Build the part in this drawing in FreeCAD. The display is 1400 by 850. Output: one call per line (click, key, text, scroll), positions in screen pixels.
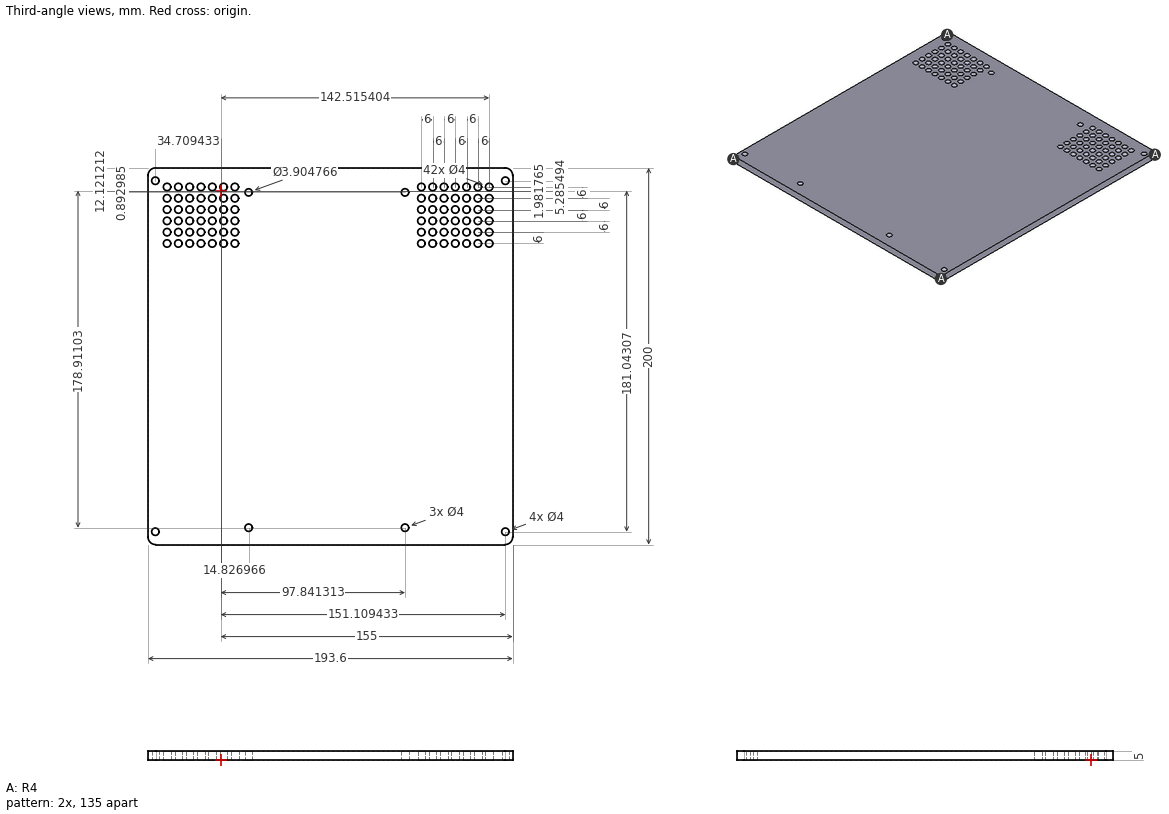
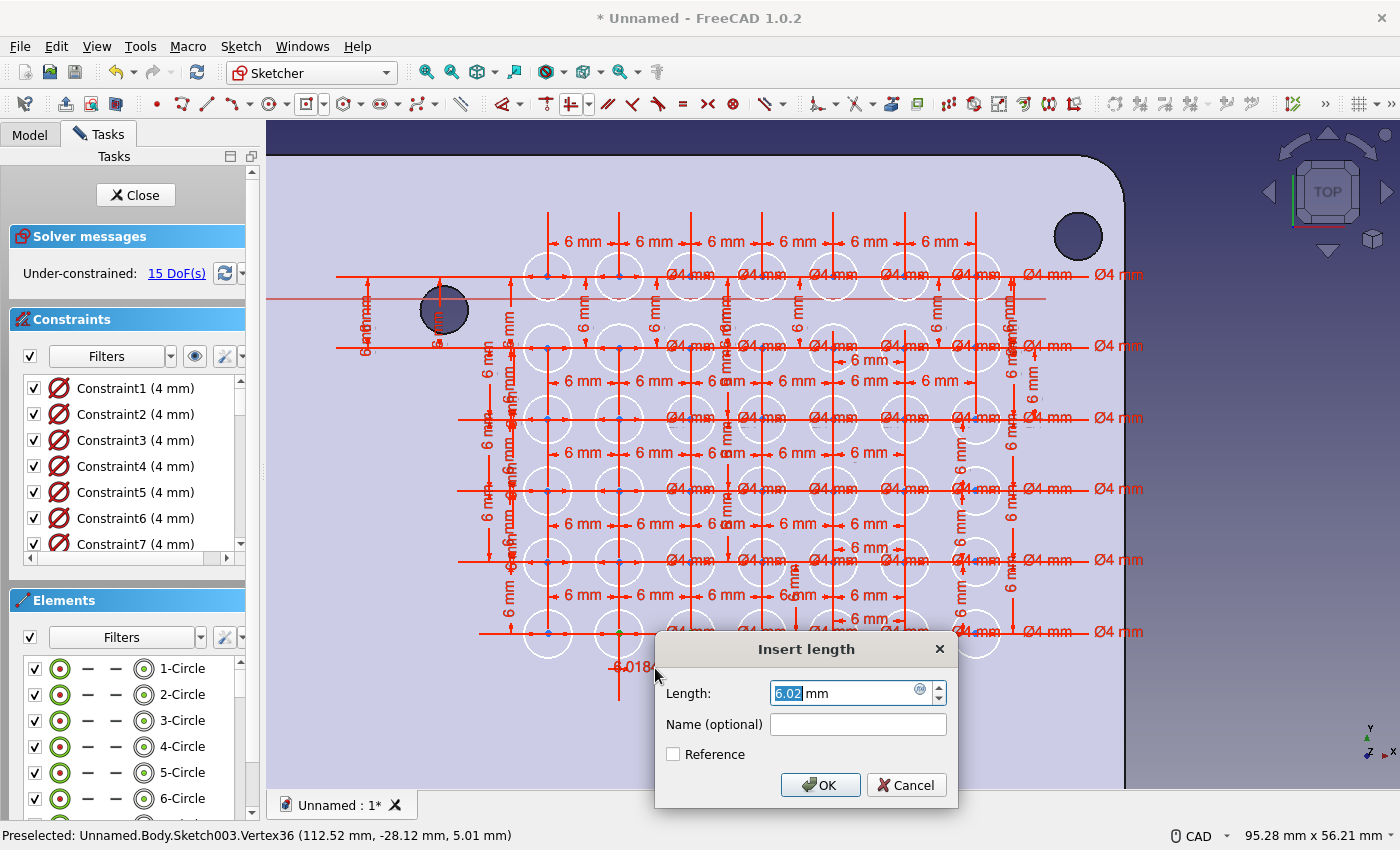
text(6)
key(Return)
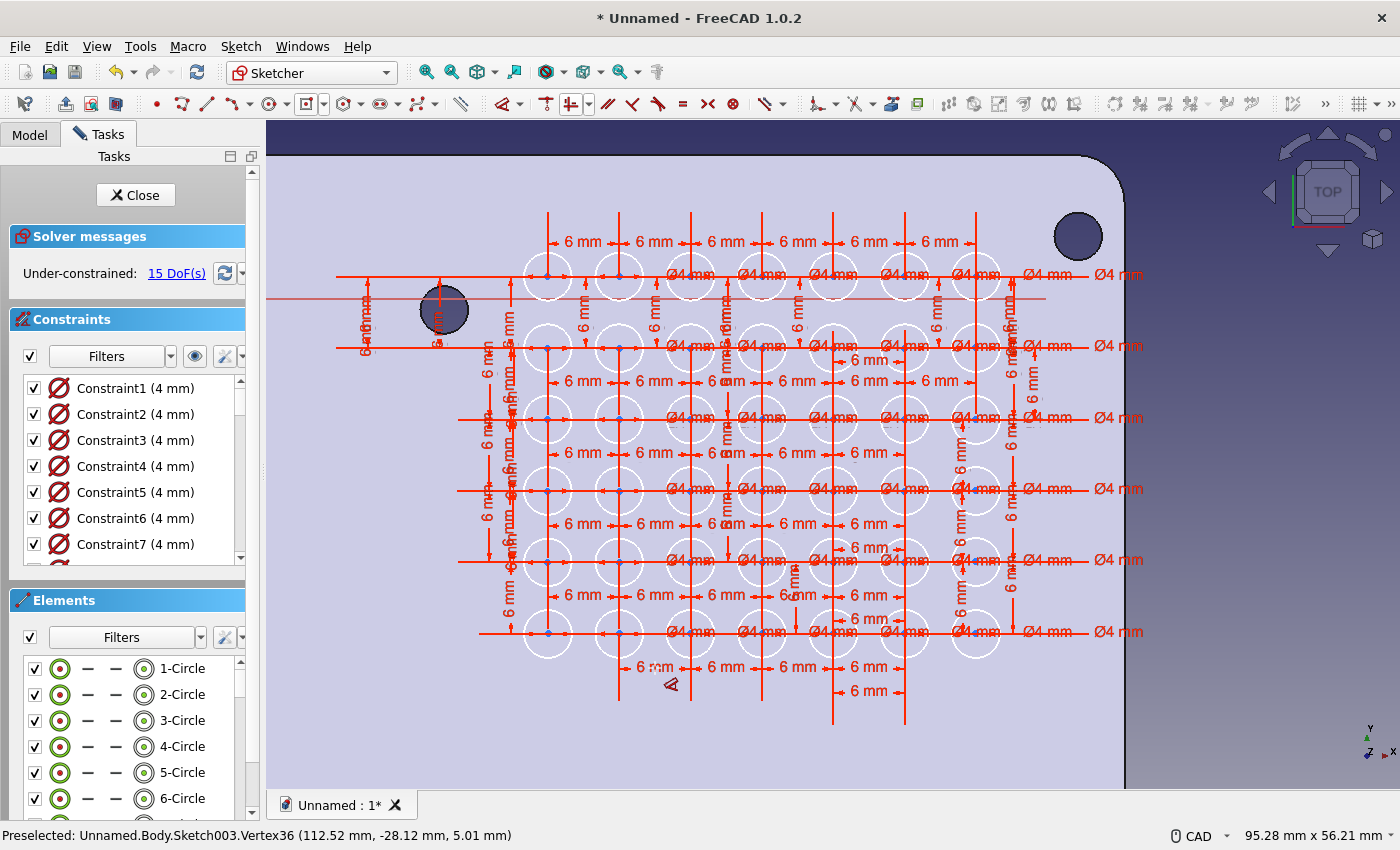
click(619, 562)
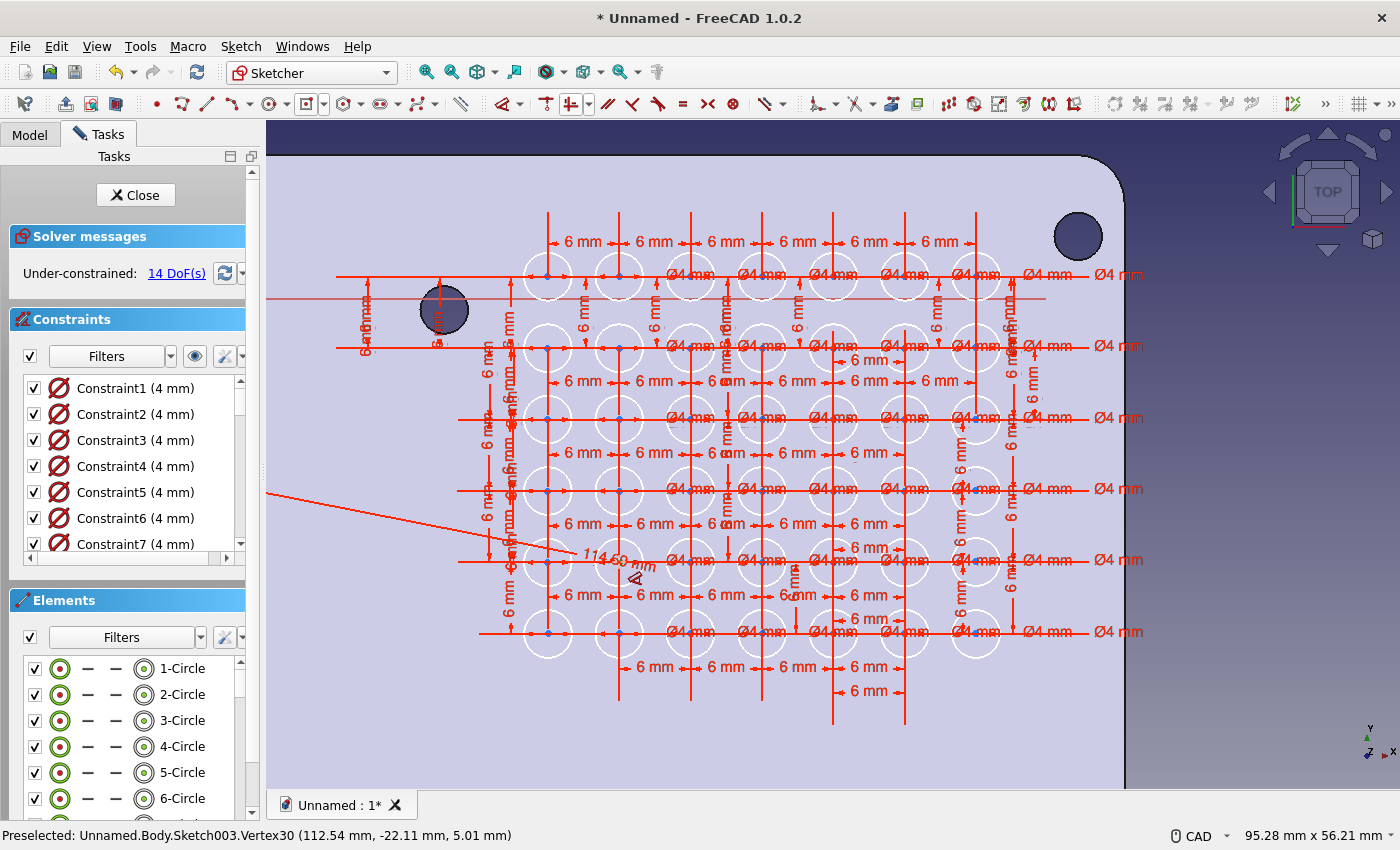
click(619, 634)
click(489, 573)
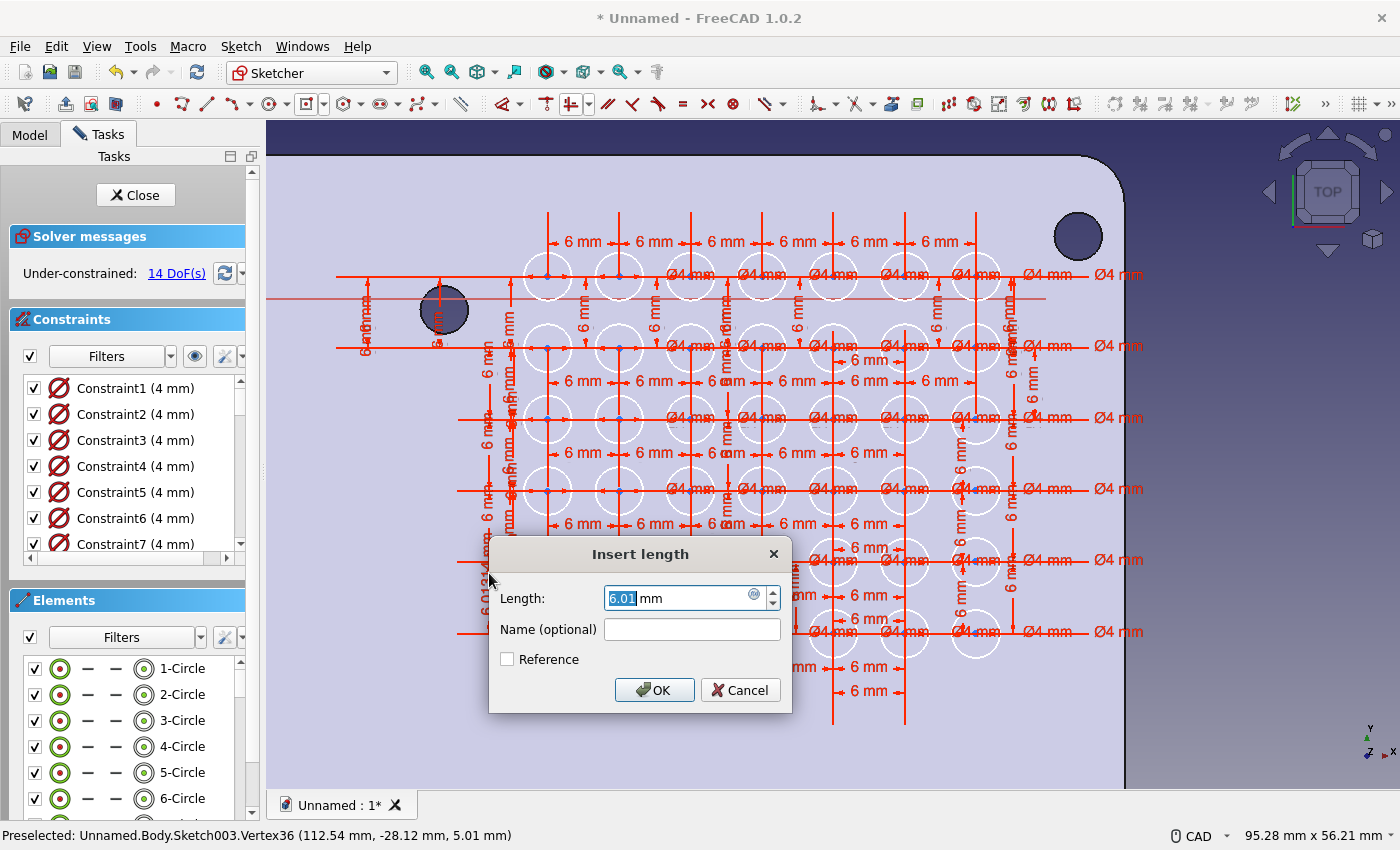
text(6)
key(Return)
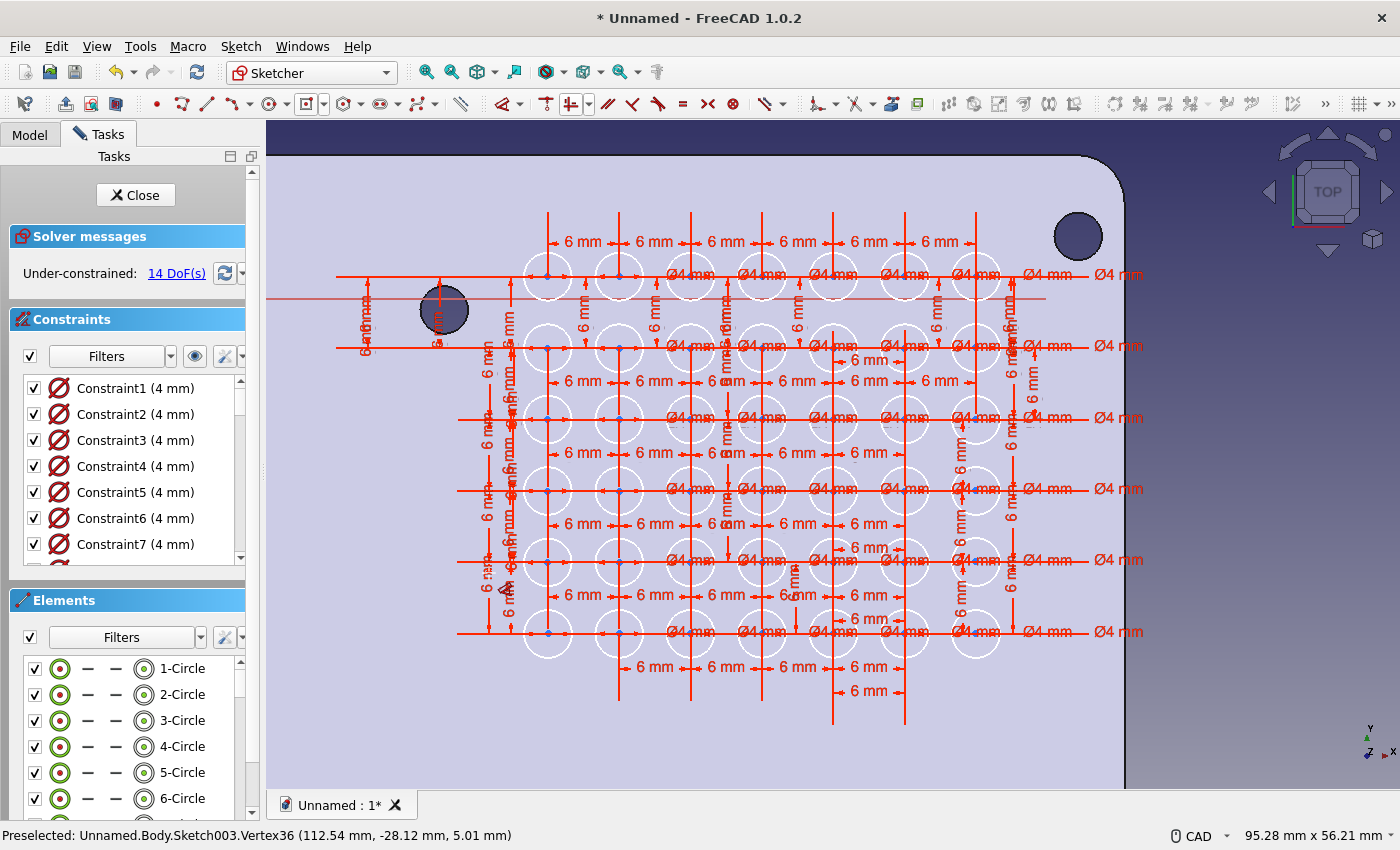
click(619, 634)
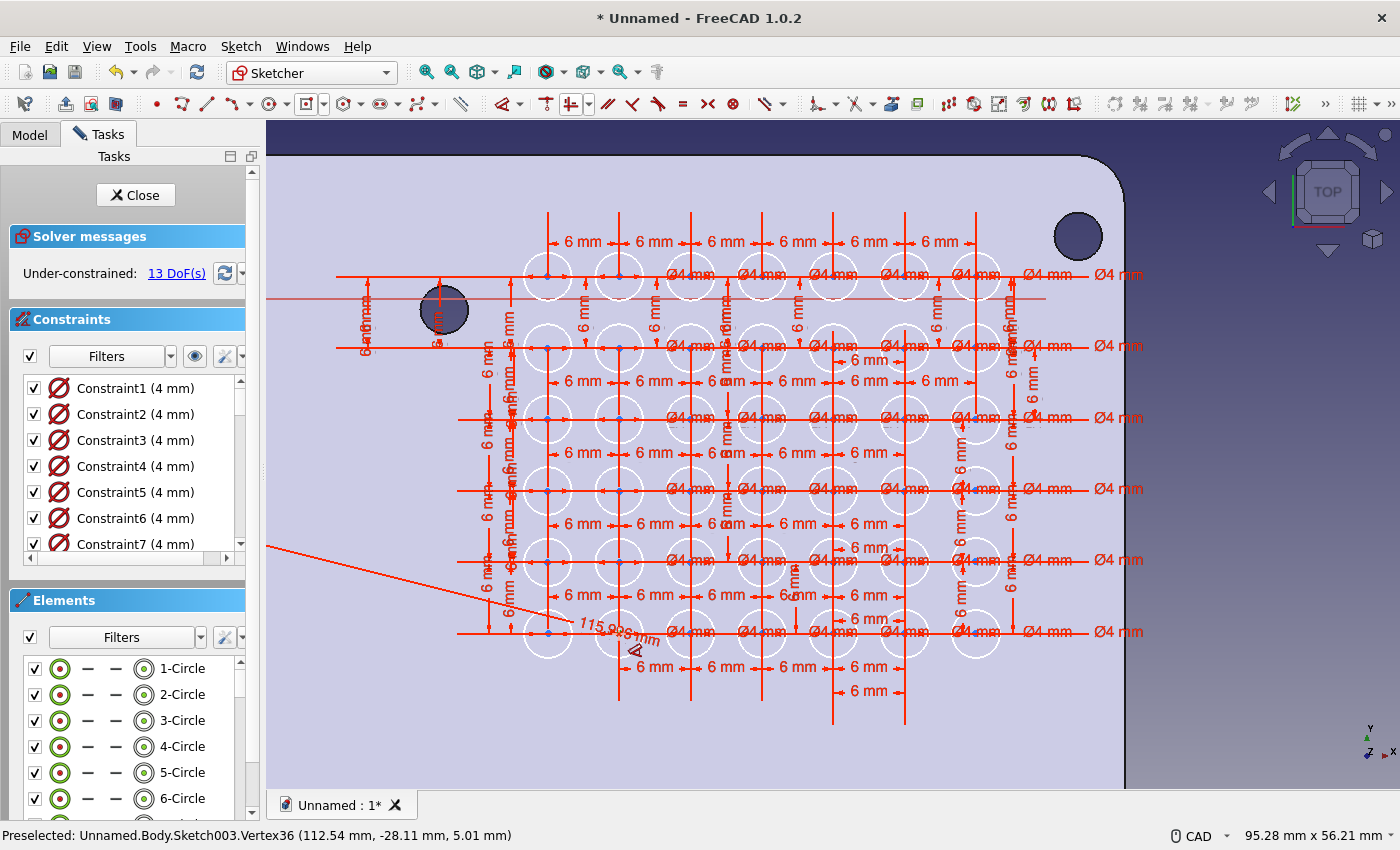
click(548, 634)
click(584, 668)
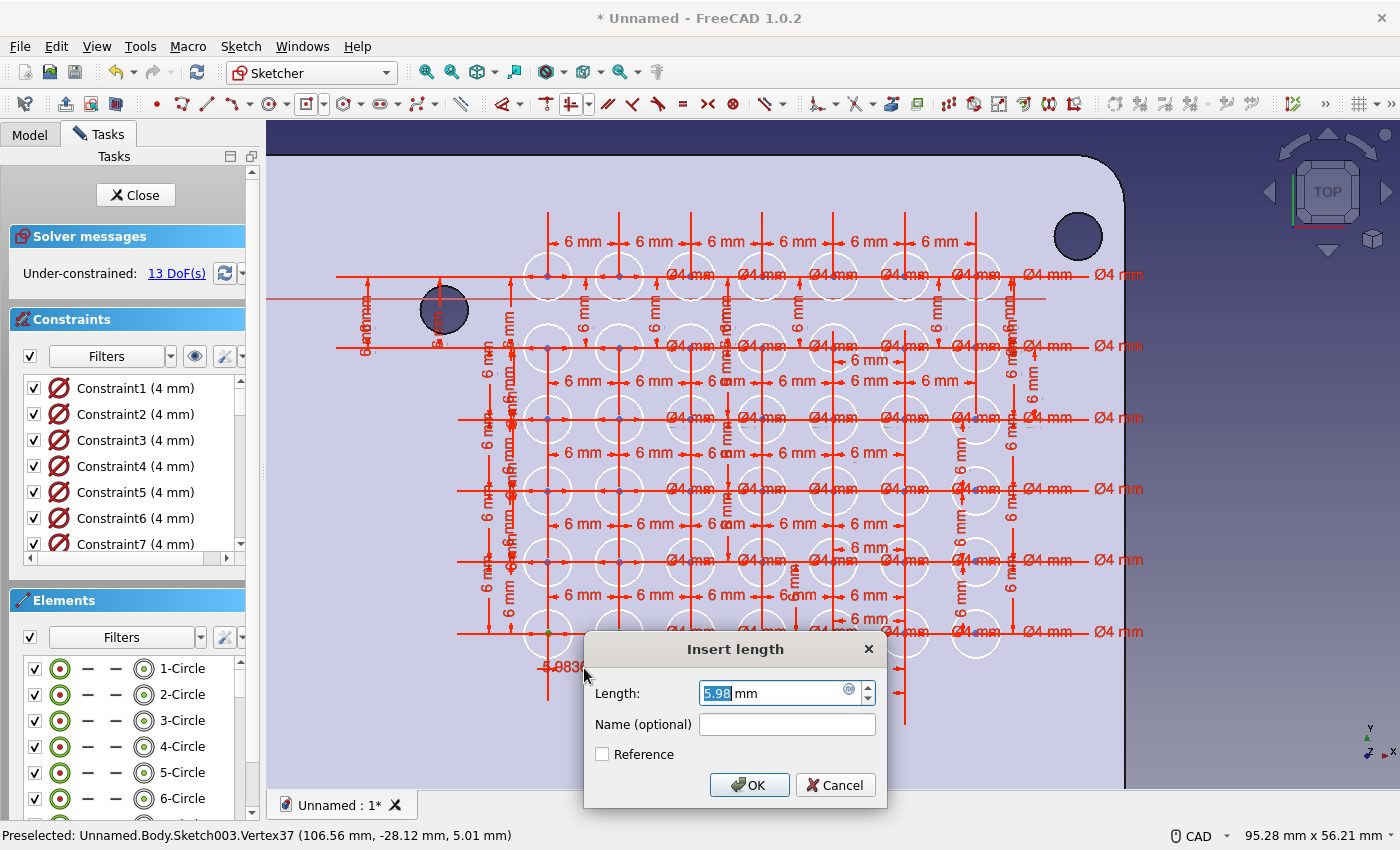
text(6)
key(Return)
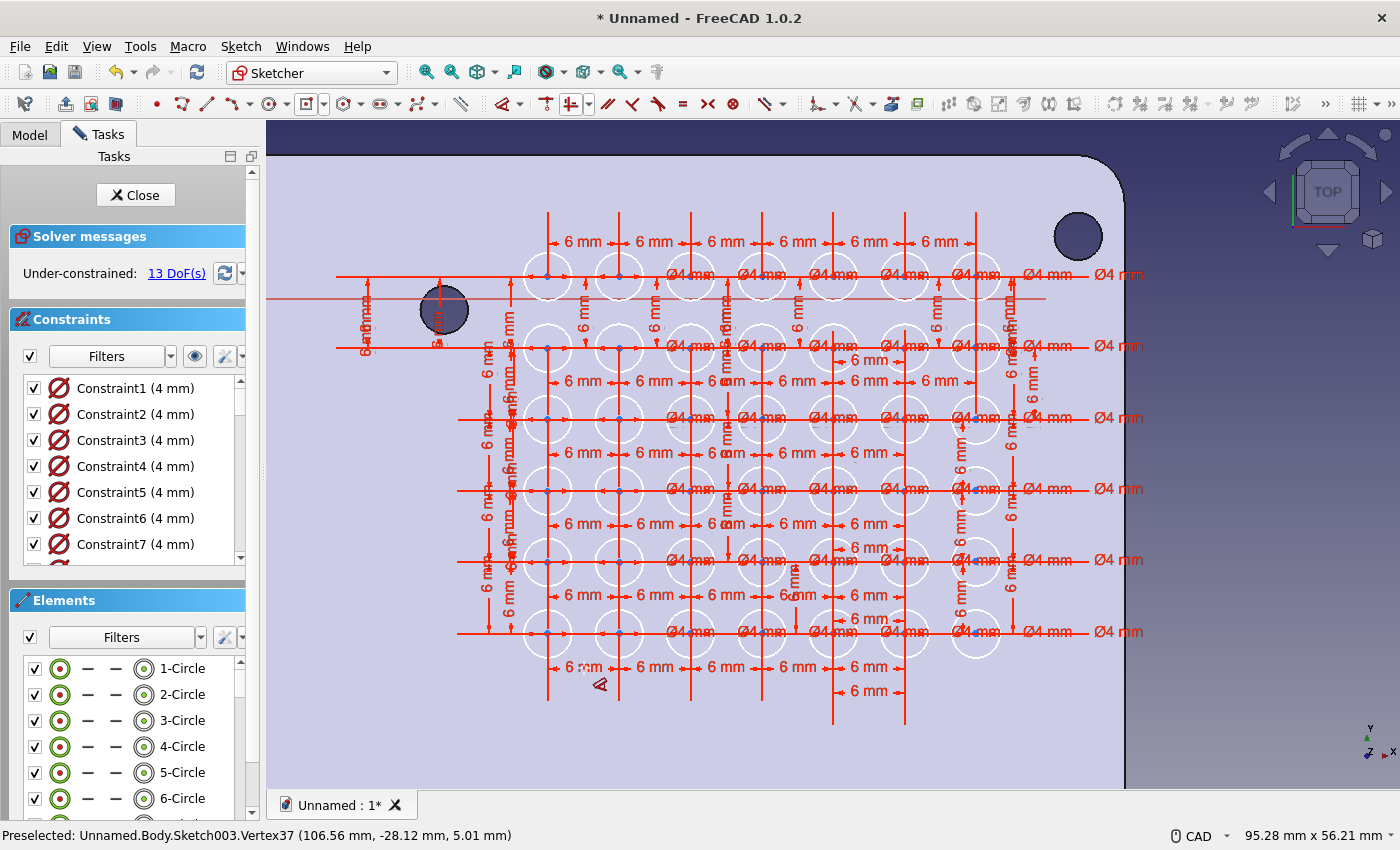
click(548, 562)